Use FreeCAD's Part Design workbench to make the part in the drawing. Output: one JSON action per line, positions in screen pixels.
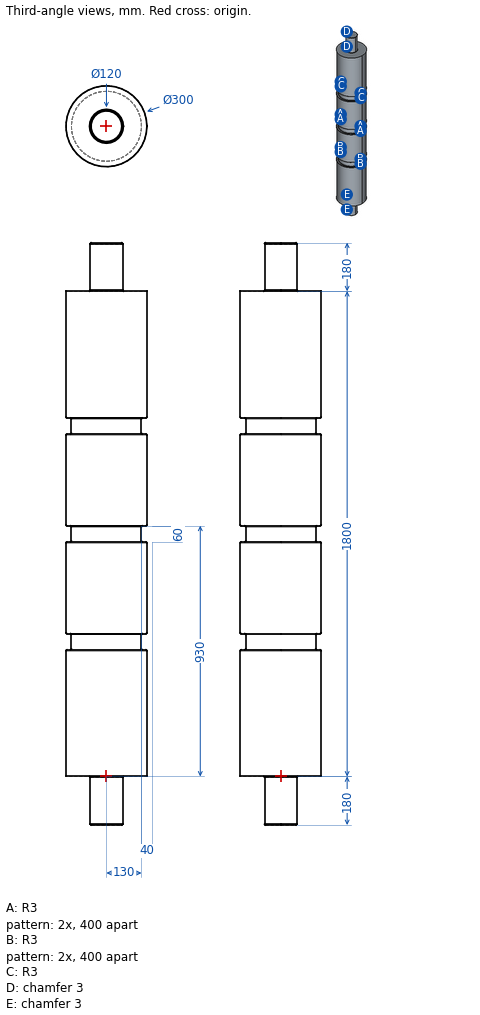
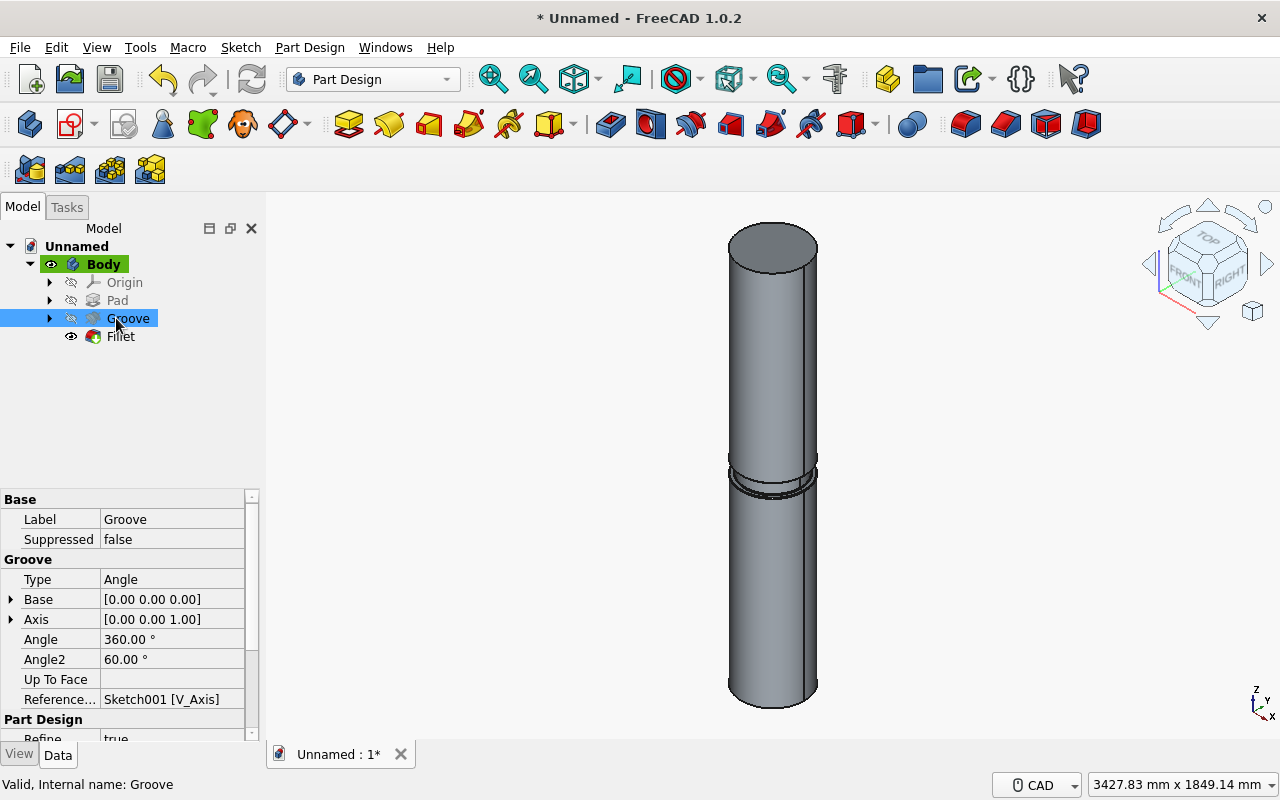
{"action": "left_click", "coordinate": [70, 170]}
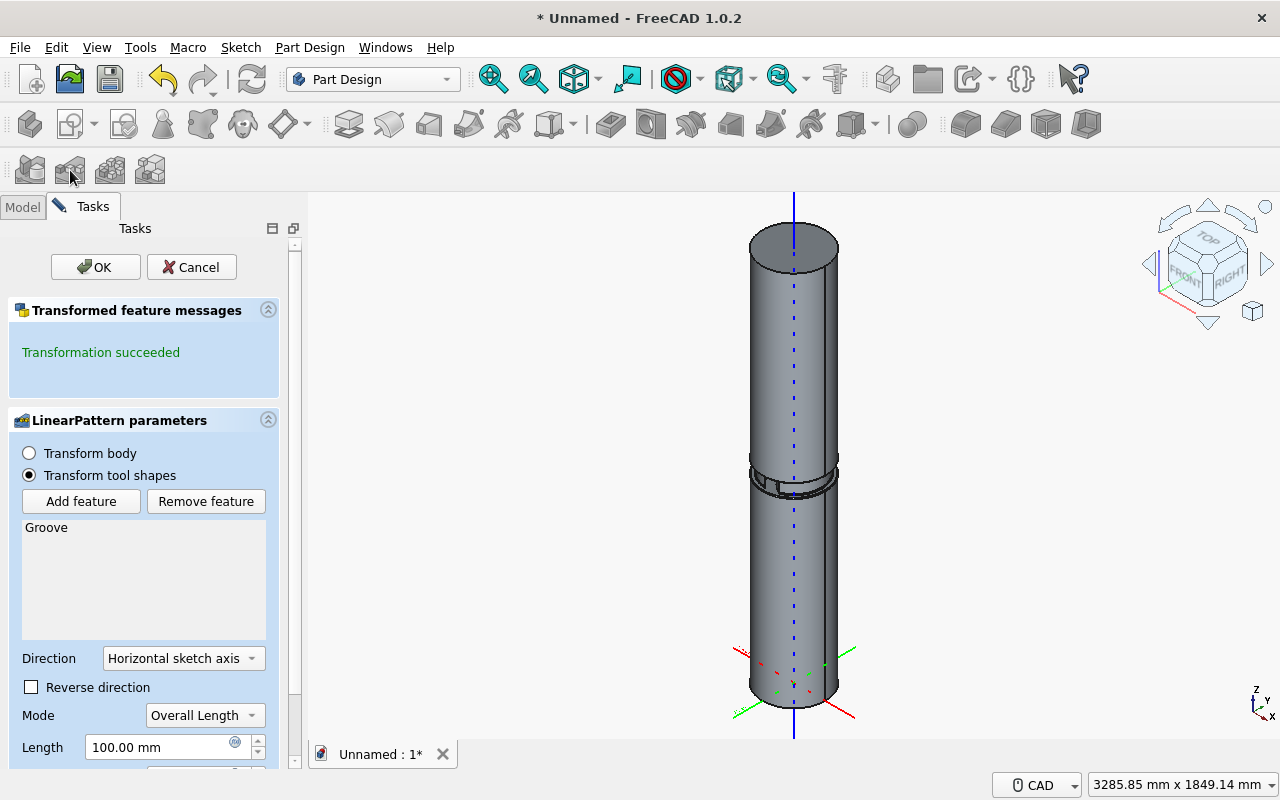
{"action": "left_click", "coordinate": [184, 658]}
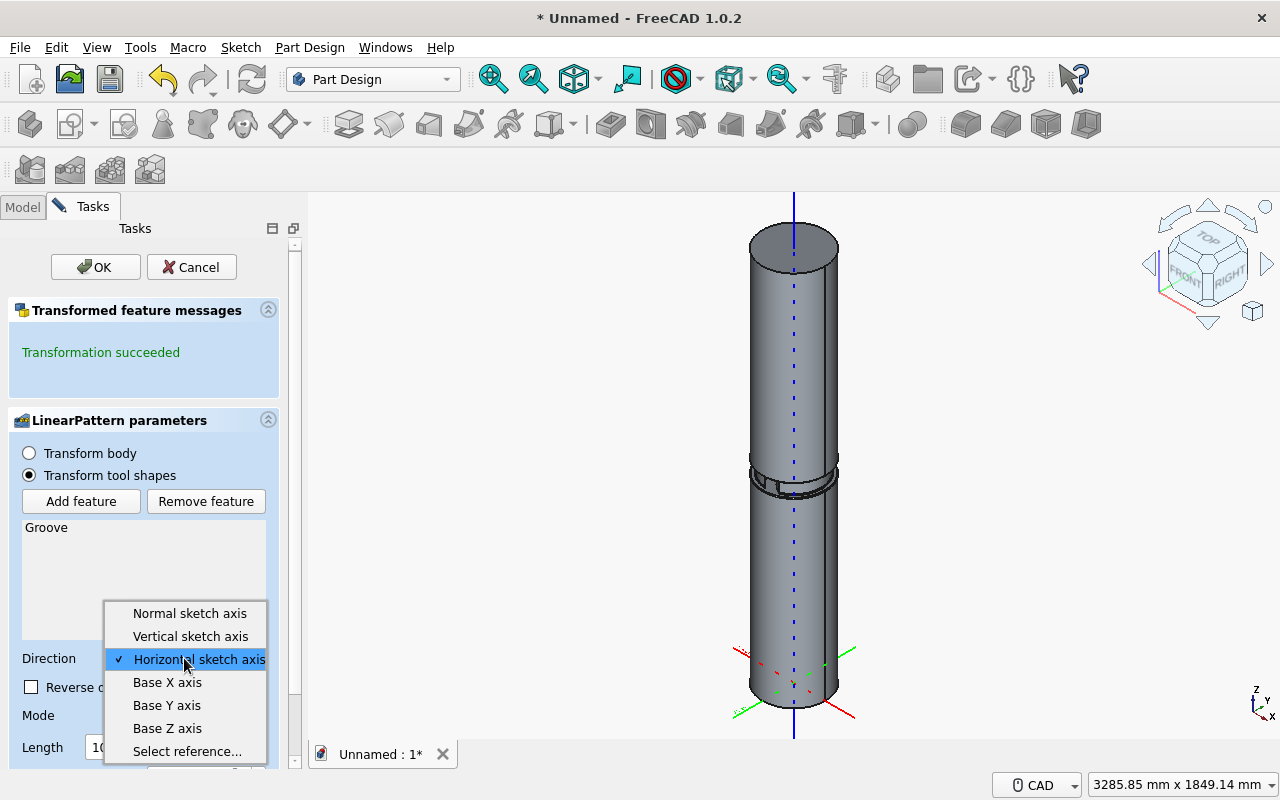
{"action": "left_click", "coordinate": [184, 728]}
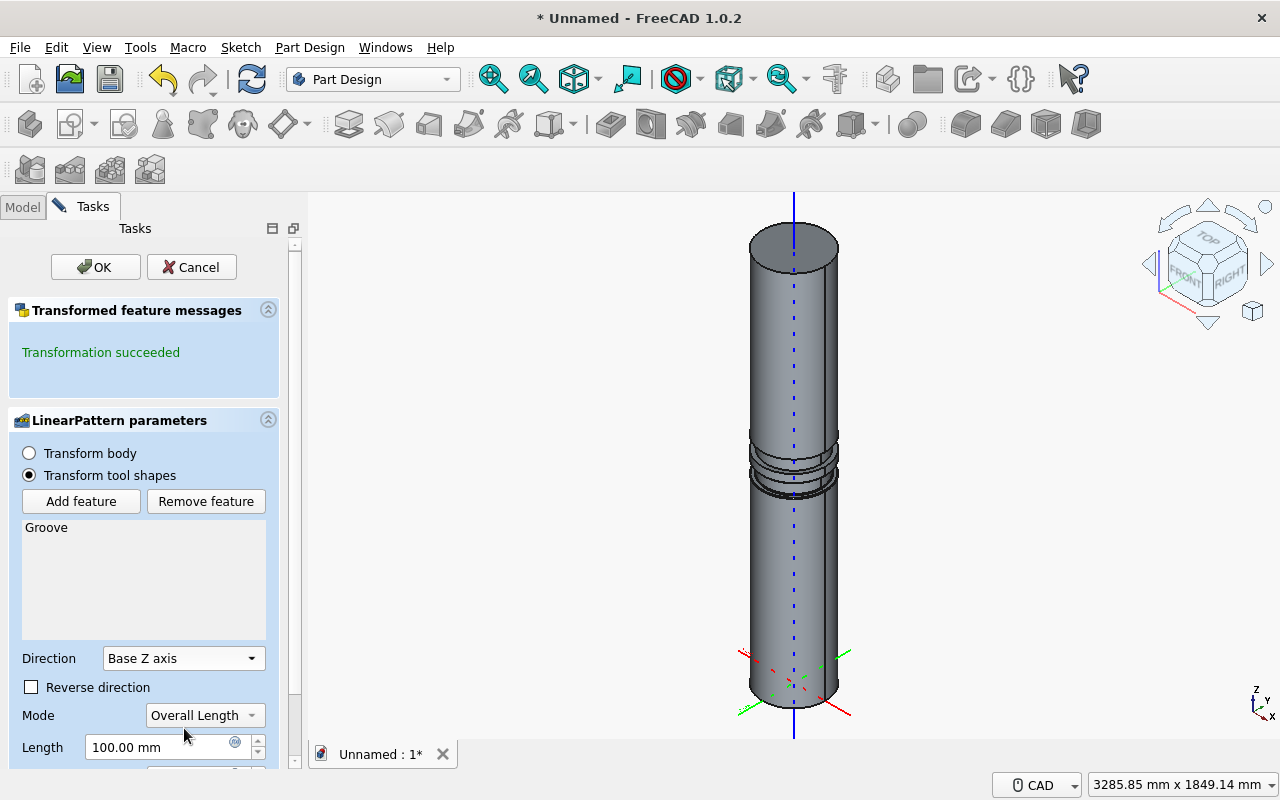
{"action": "left_click", "coordinate": [206, 716]}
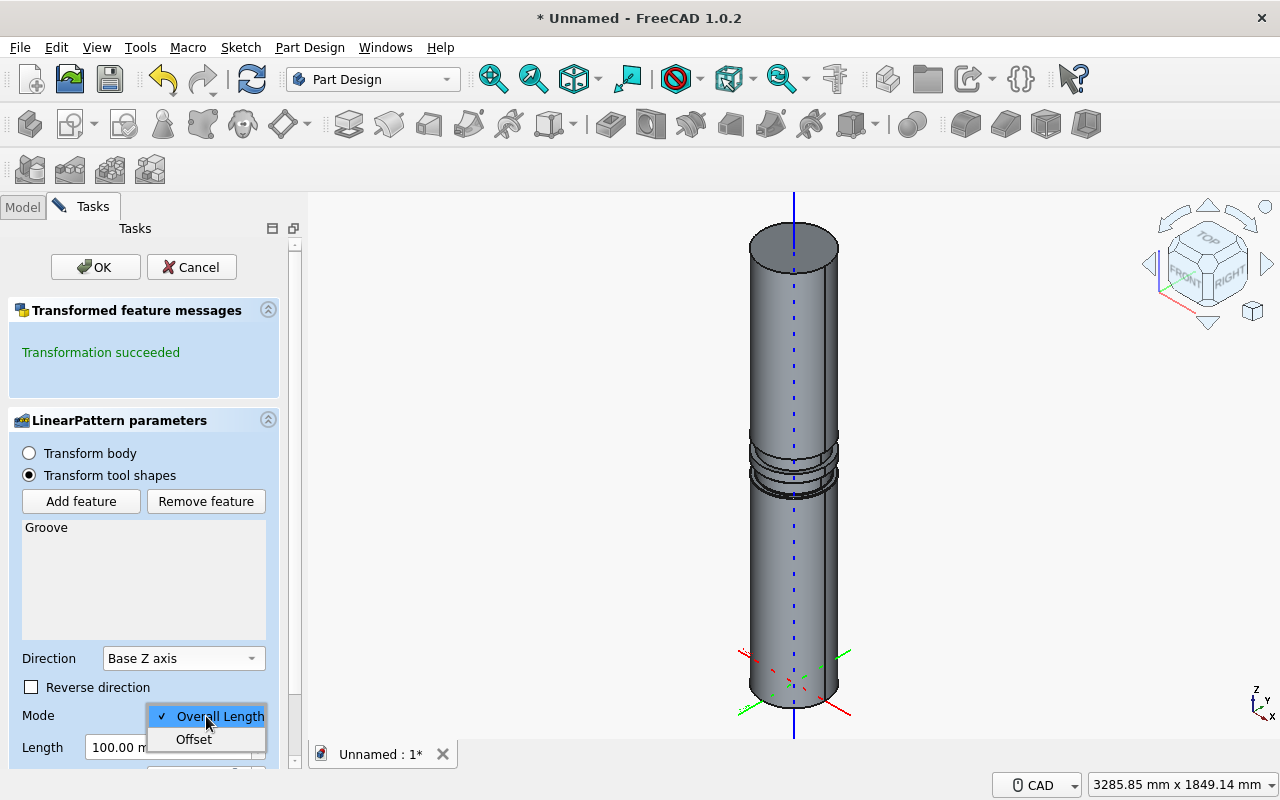
{"action": "left_click", "coordinate": [206, 740]}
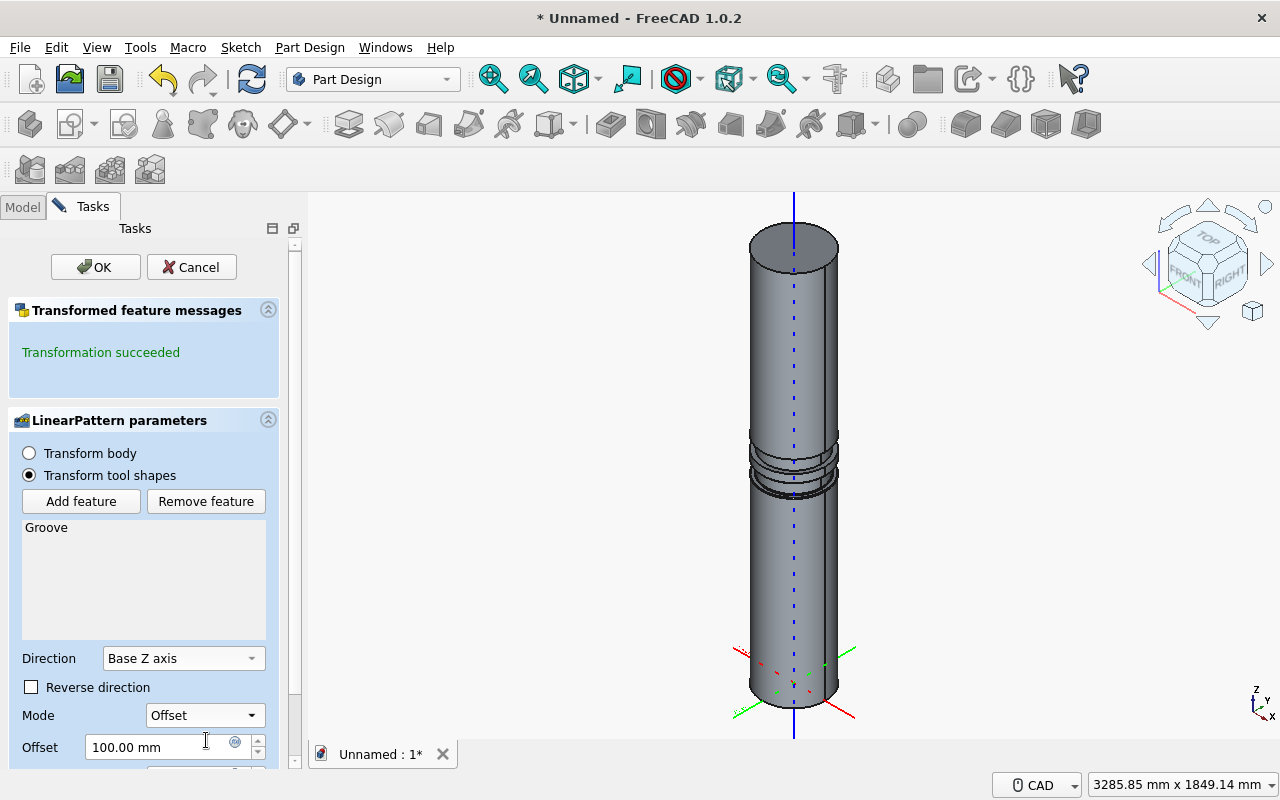
{"action": "triple_click", "coordinate": [168, 747]}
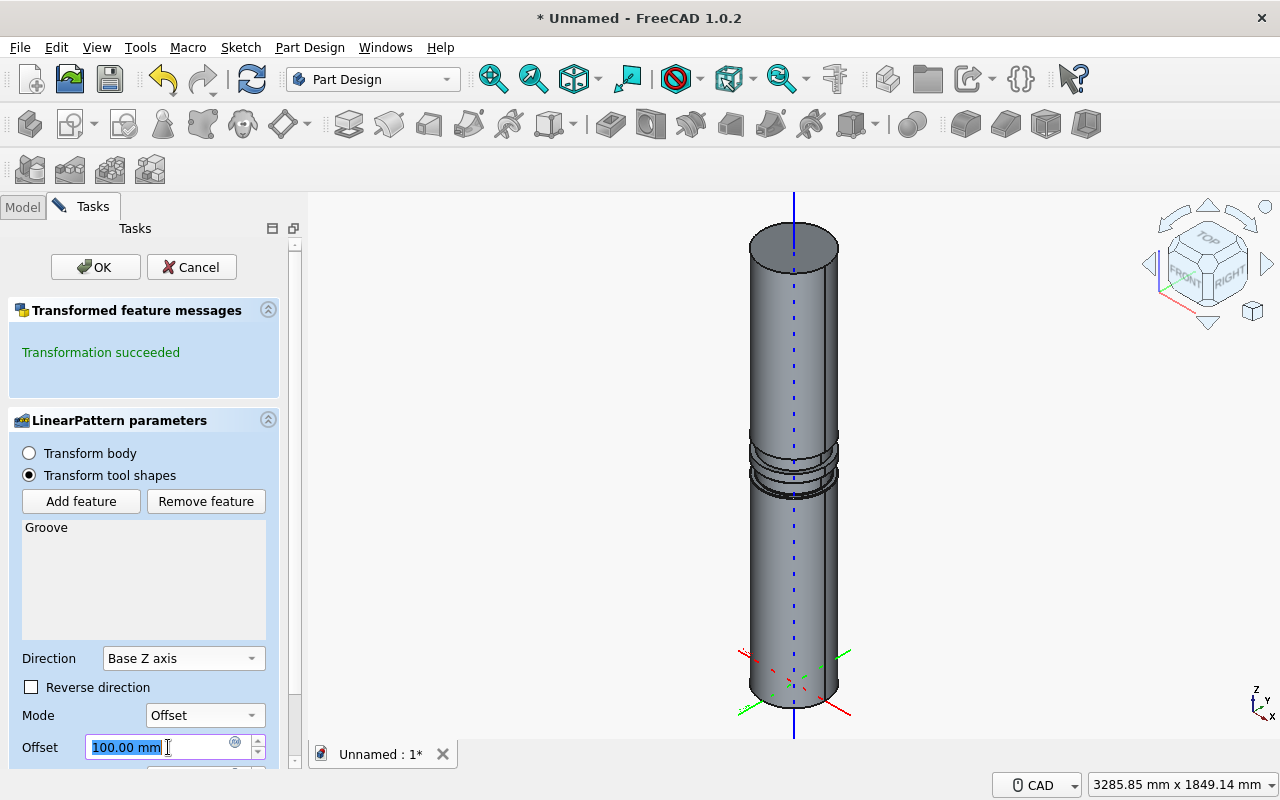
{"action": "type", "text": "400"}
{"action": "key", "text": "Tab"}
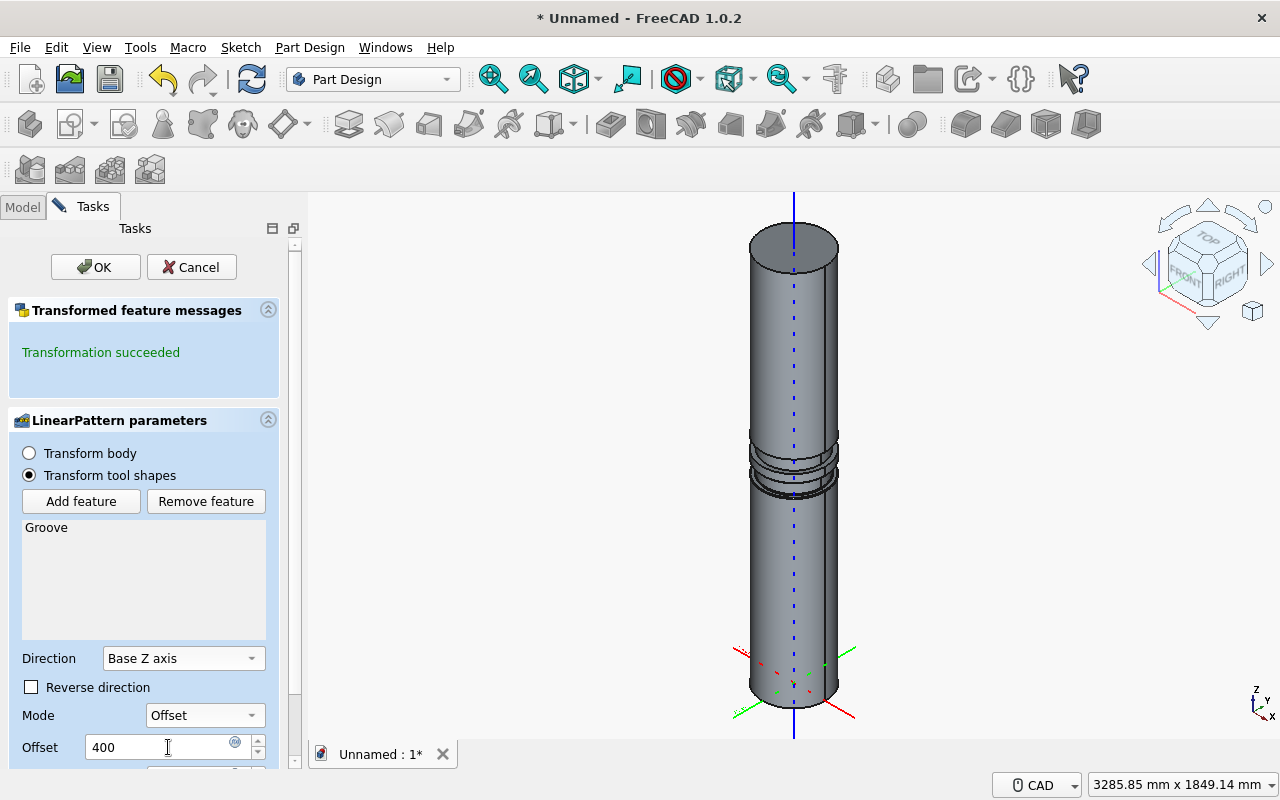
{"action": "scroll", "coordinate": [295, 503], "scroll_direction": "down", "scroll_amount": 2}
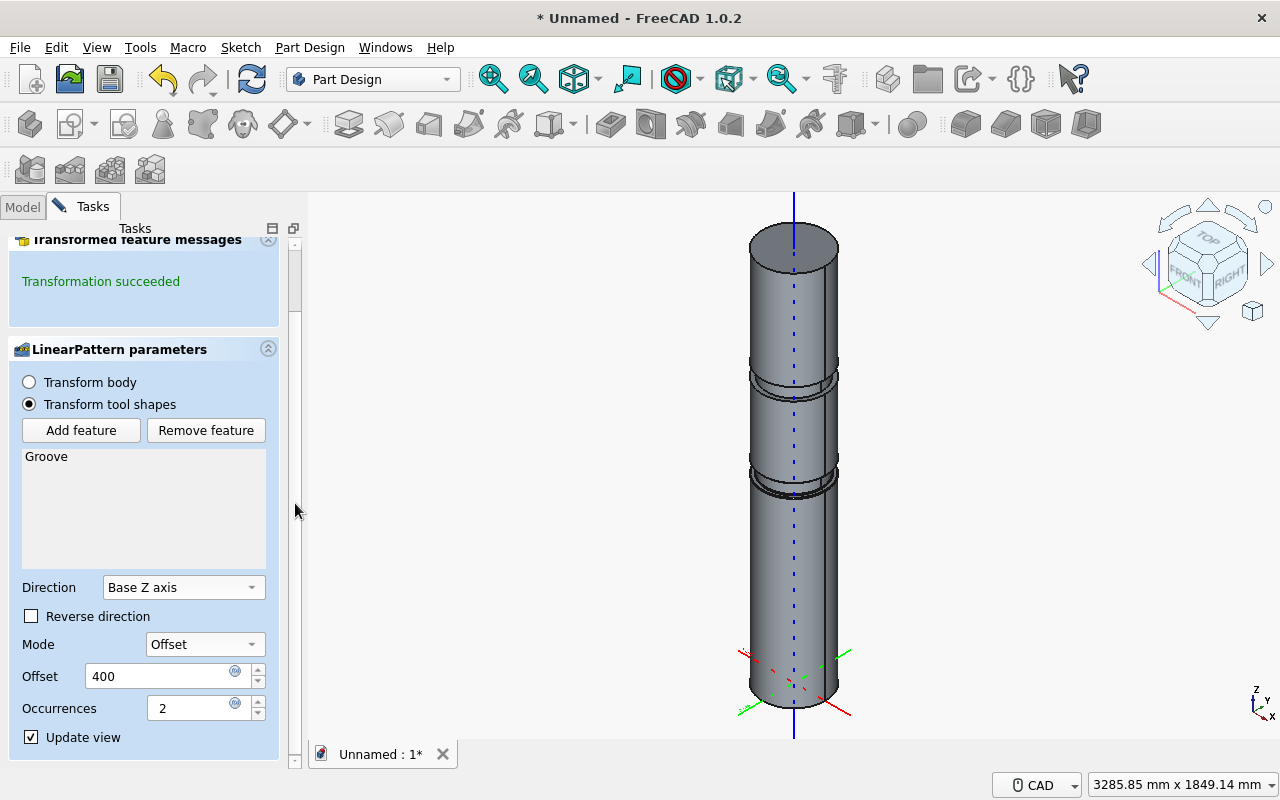
{"action": "triple_click", "coordinate": [198, 708]}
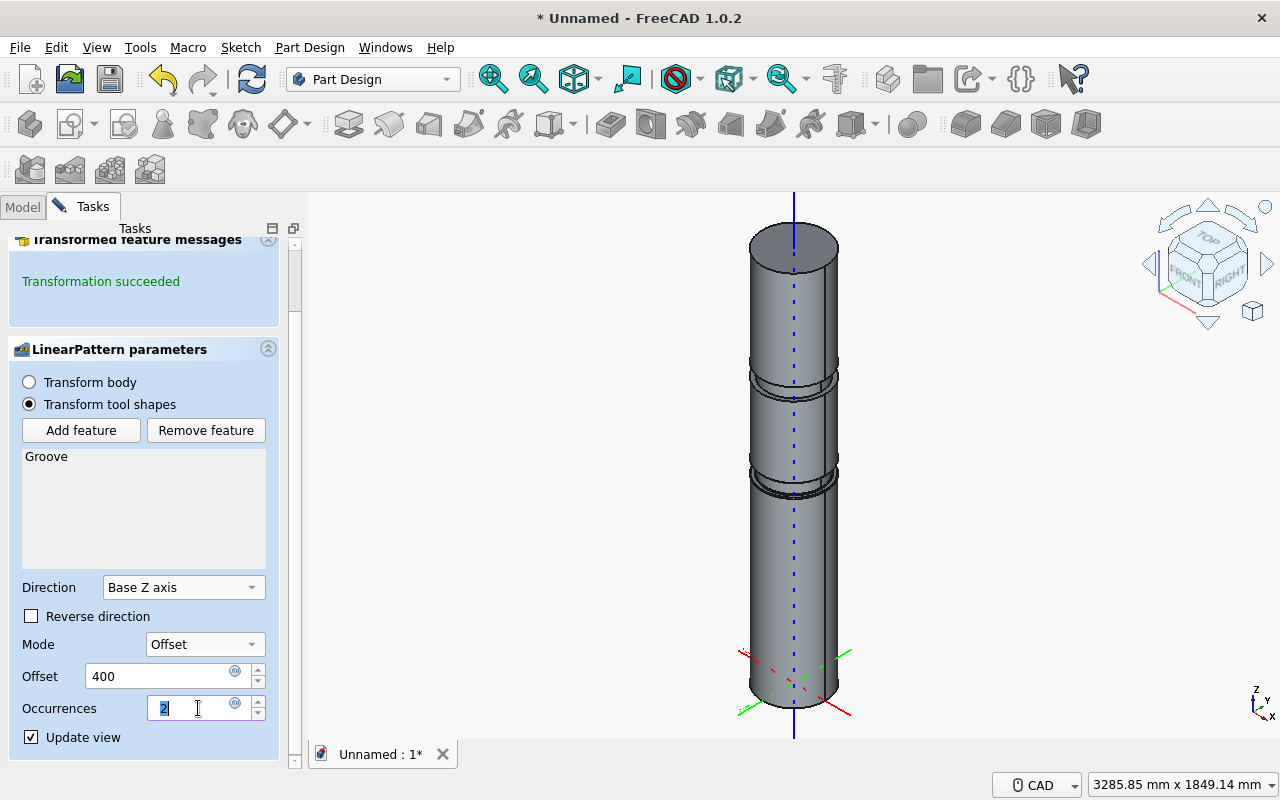
{"action": "type", "text": "2"}
{"action": "key", "text": "Tab"}